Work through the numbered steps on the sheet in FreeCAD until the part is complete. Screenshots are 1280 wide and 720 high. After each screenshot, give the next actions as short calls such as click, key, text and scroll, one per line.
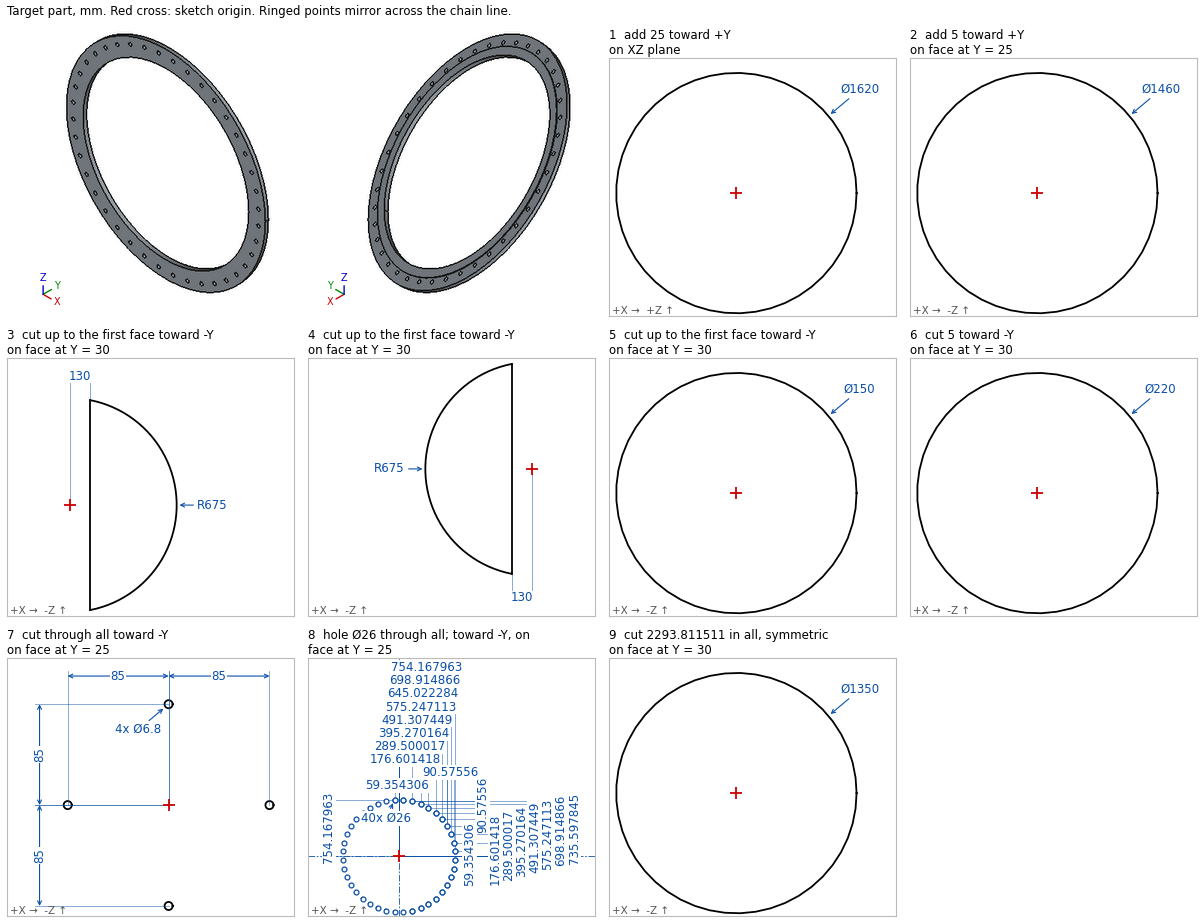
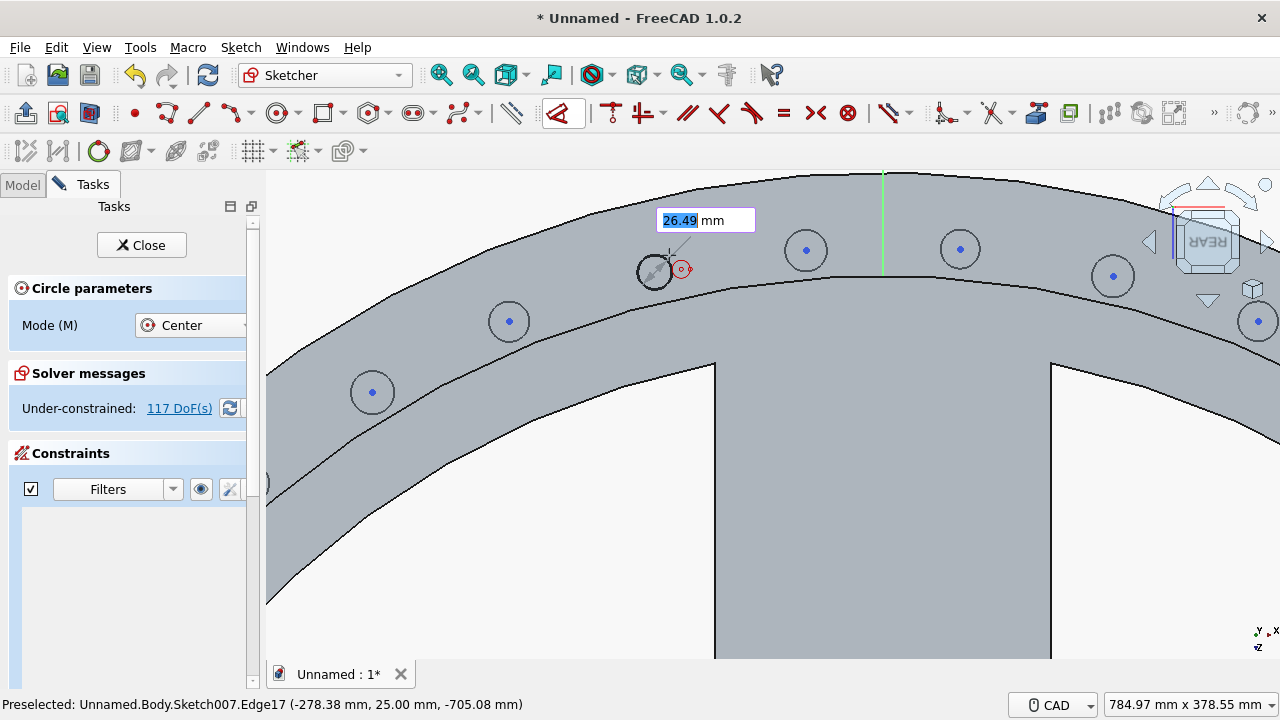
click(667, 257)
key(Escape)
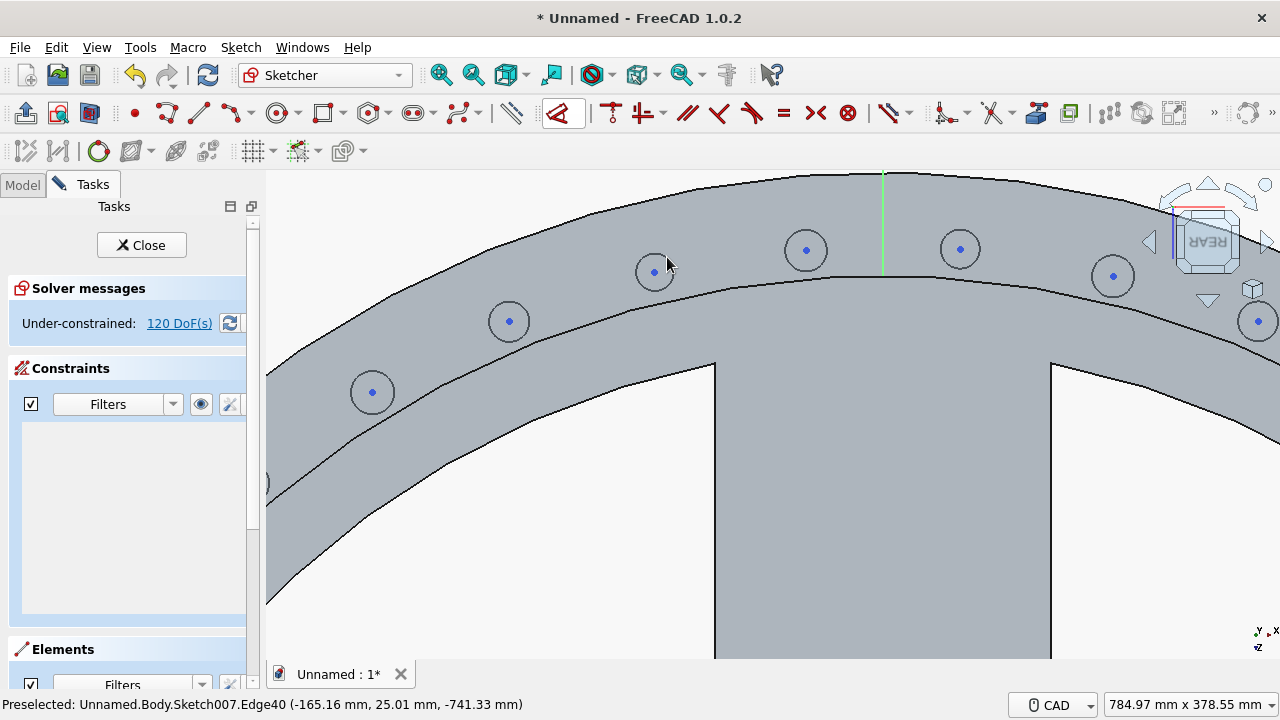
click(821, 236)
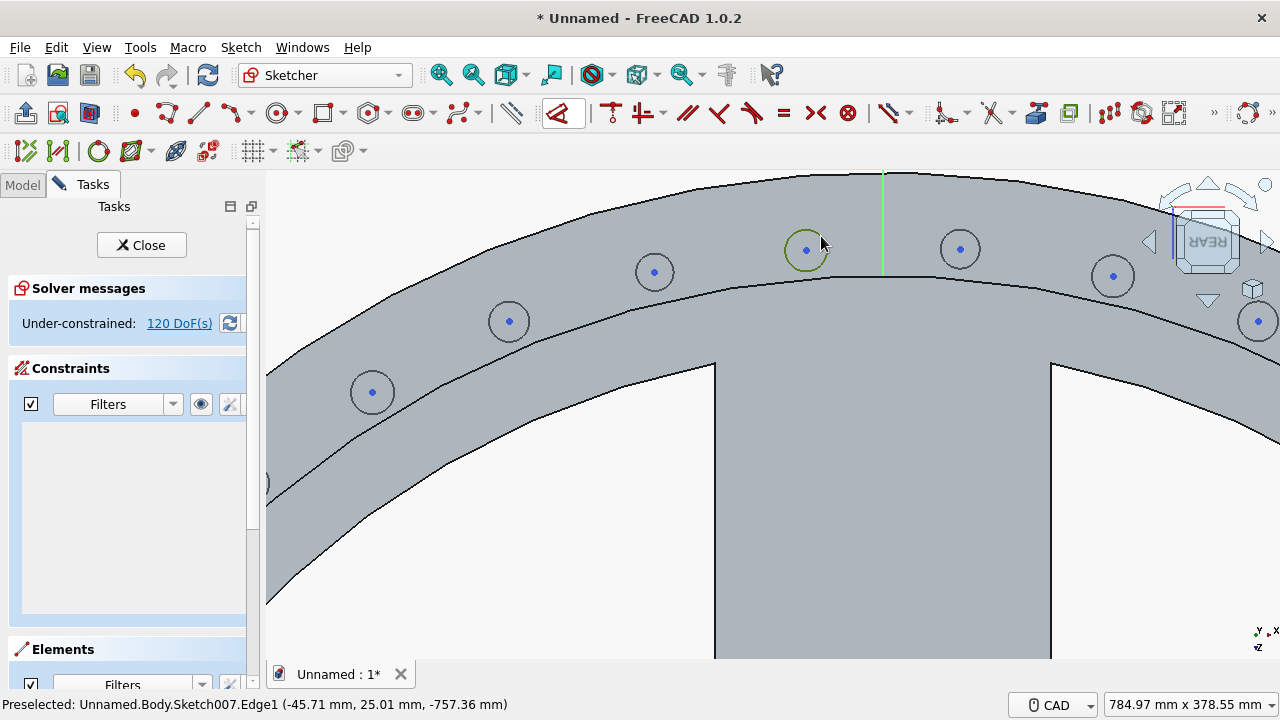
click(974, 235)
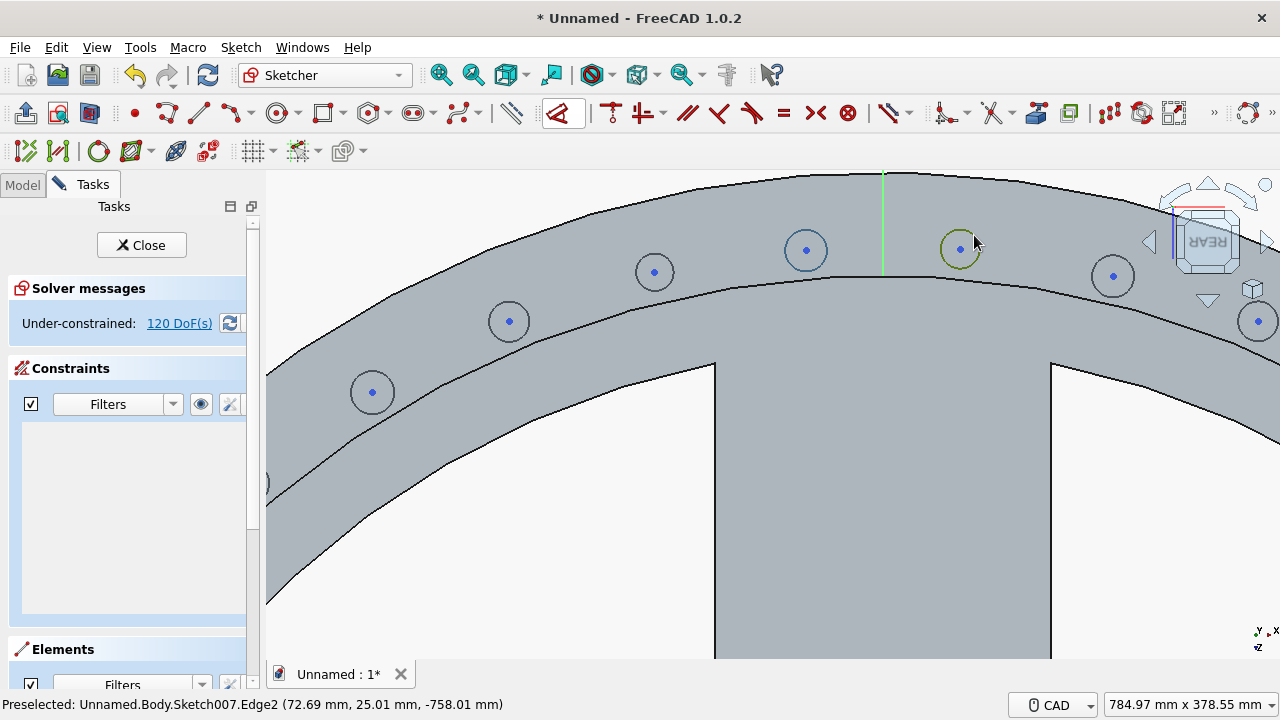
click(1098, 262)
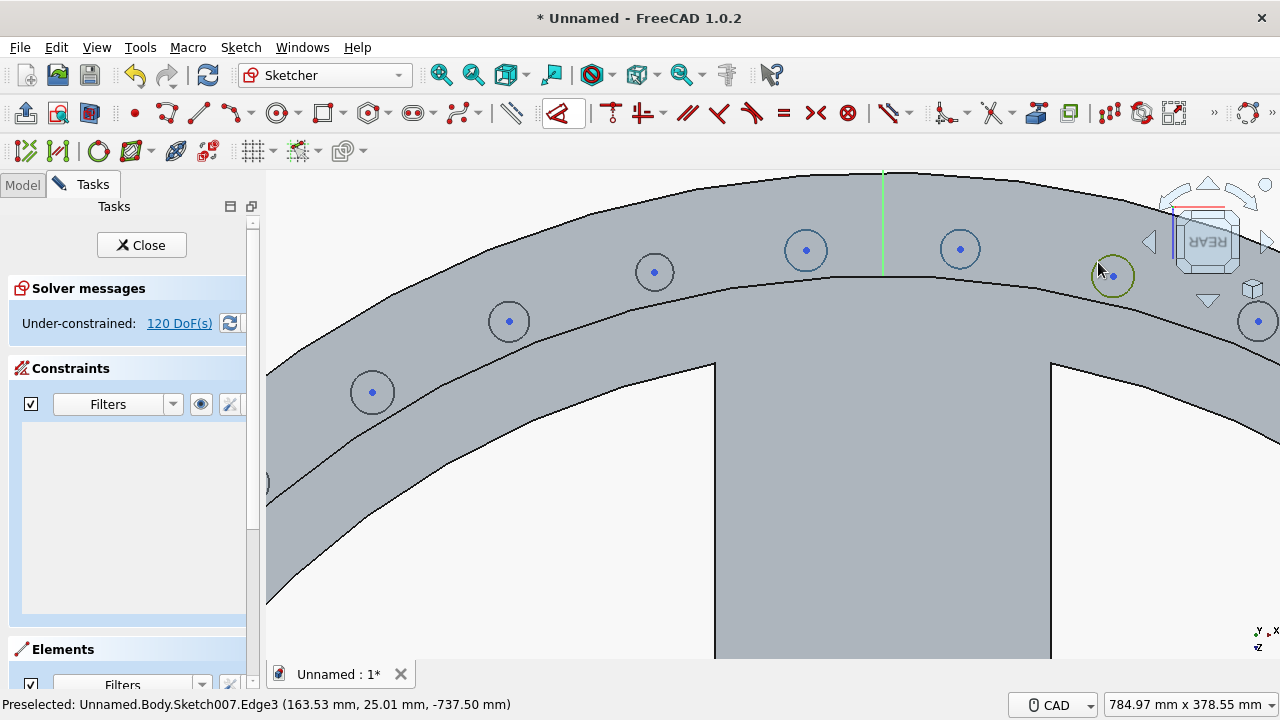
scroll(669, 255, down, 9)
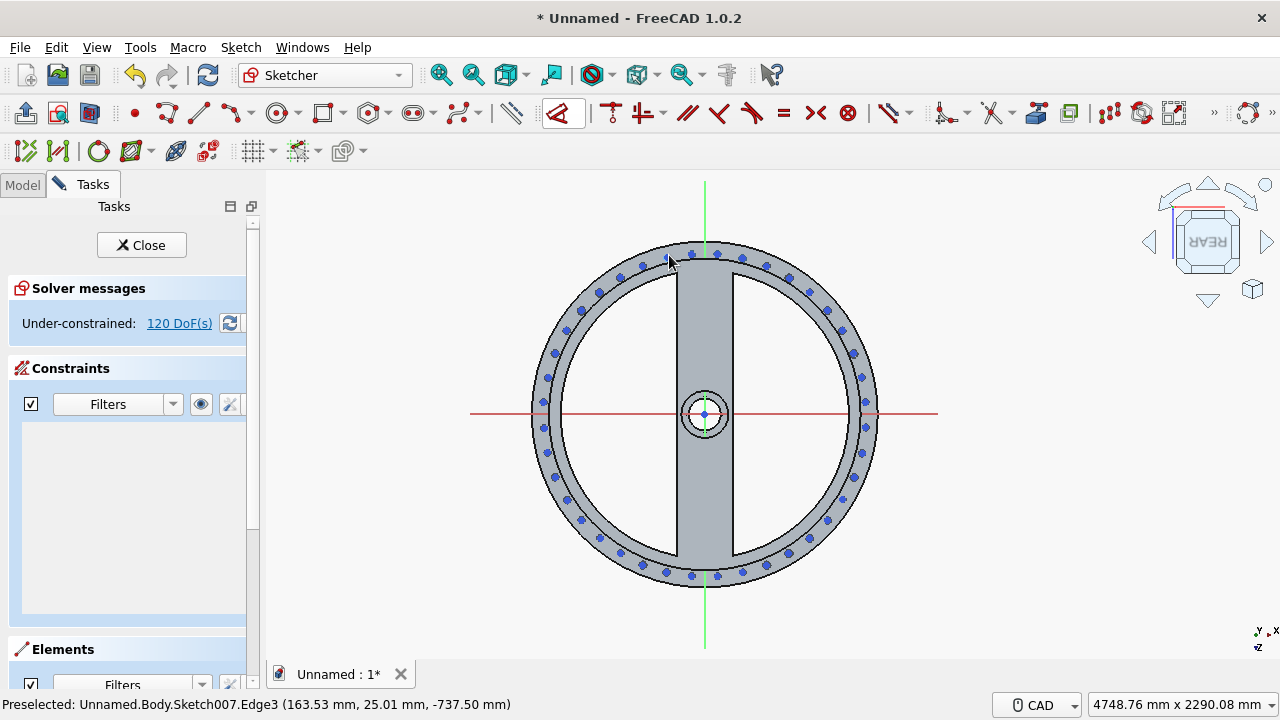
scroll(769, 264, up, 8)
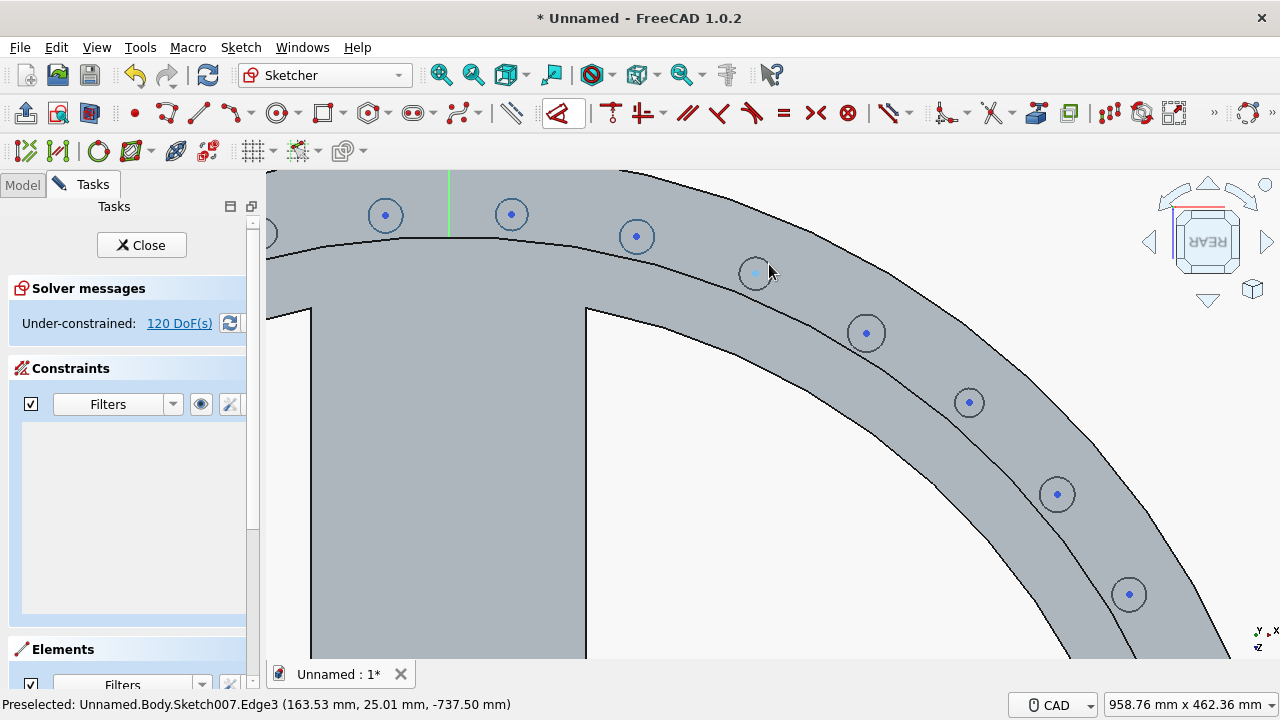
click(767, 262)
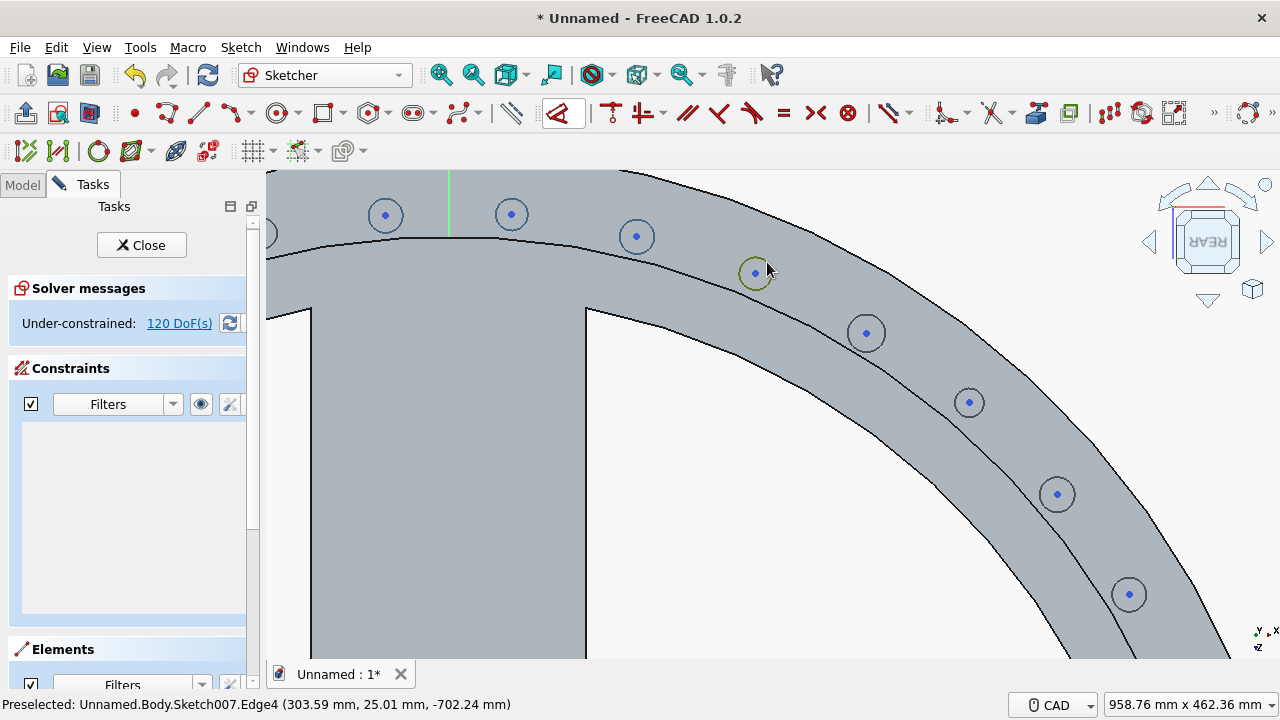
click(880, 320)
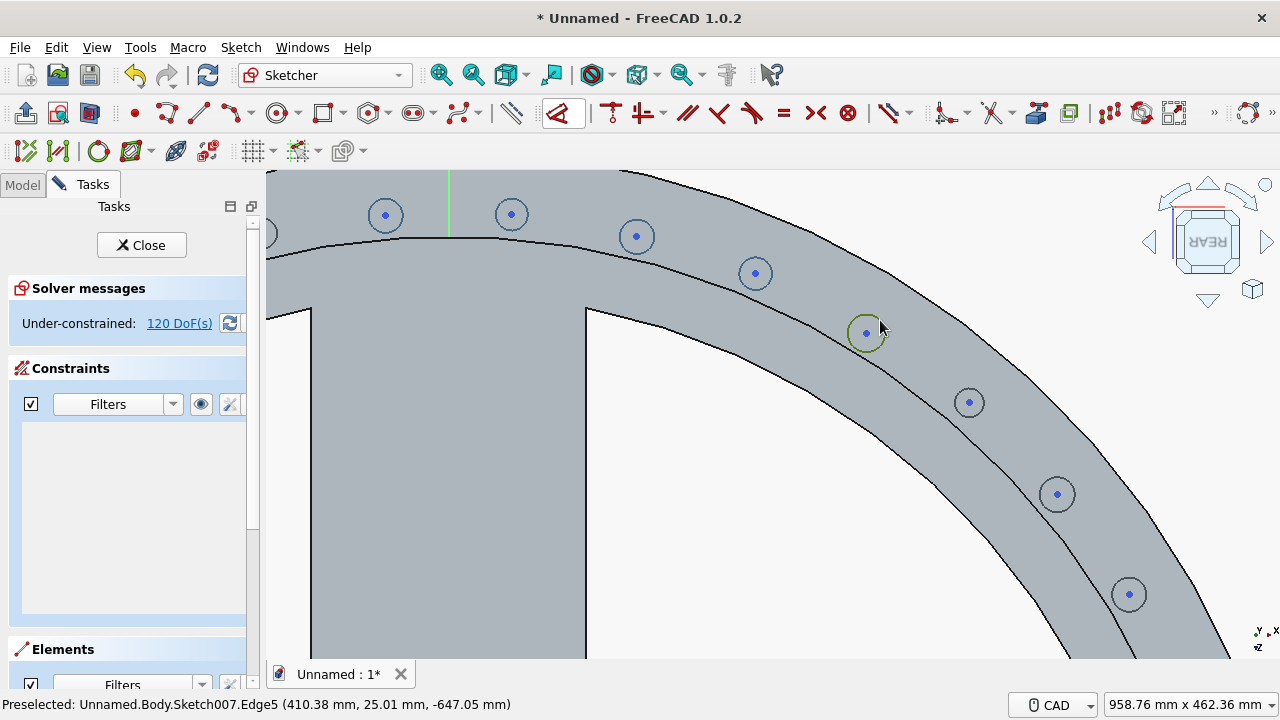
click(980, 393)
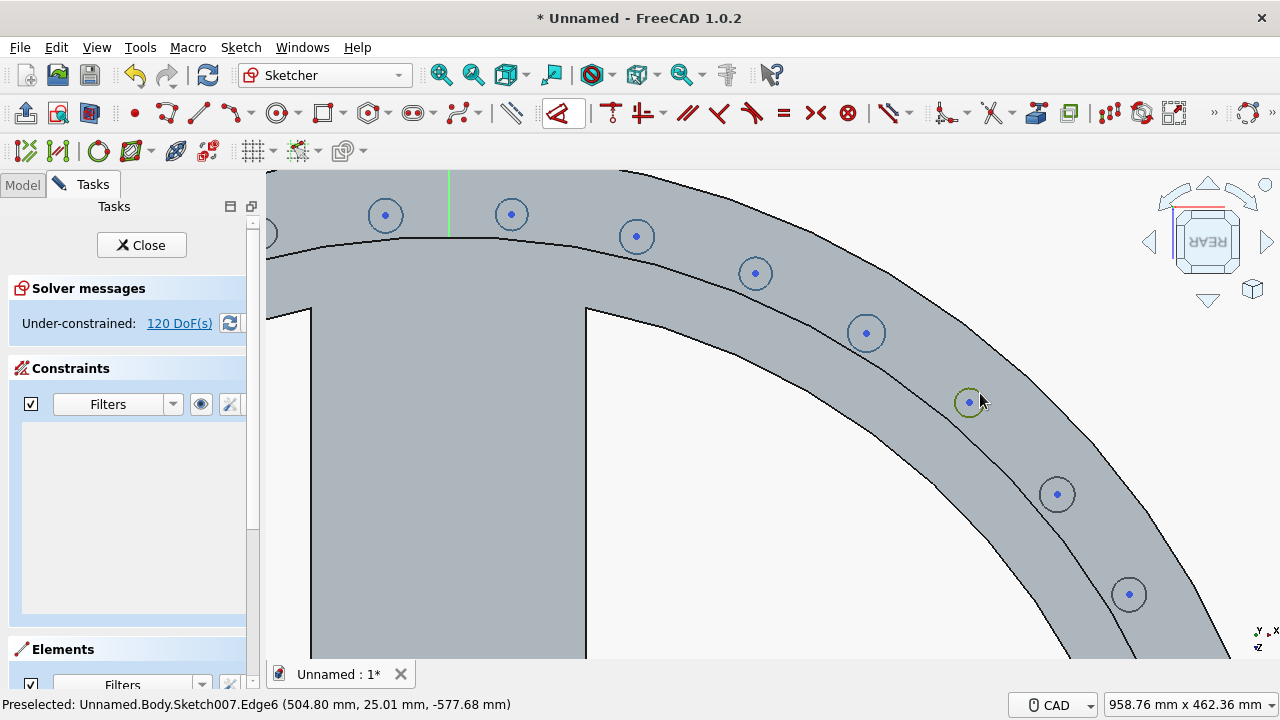
click(1070, 482)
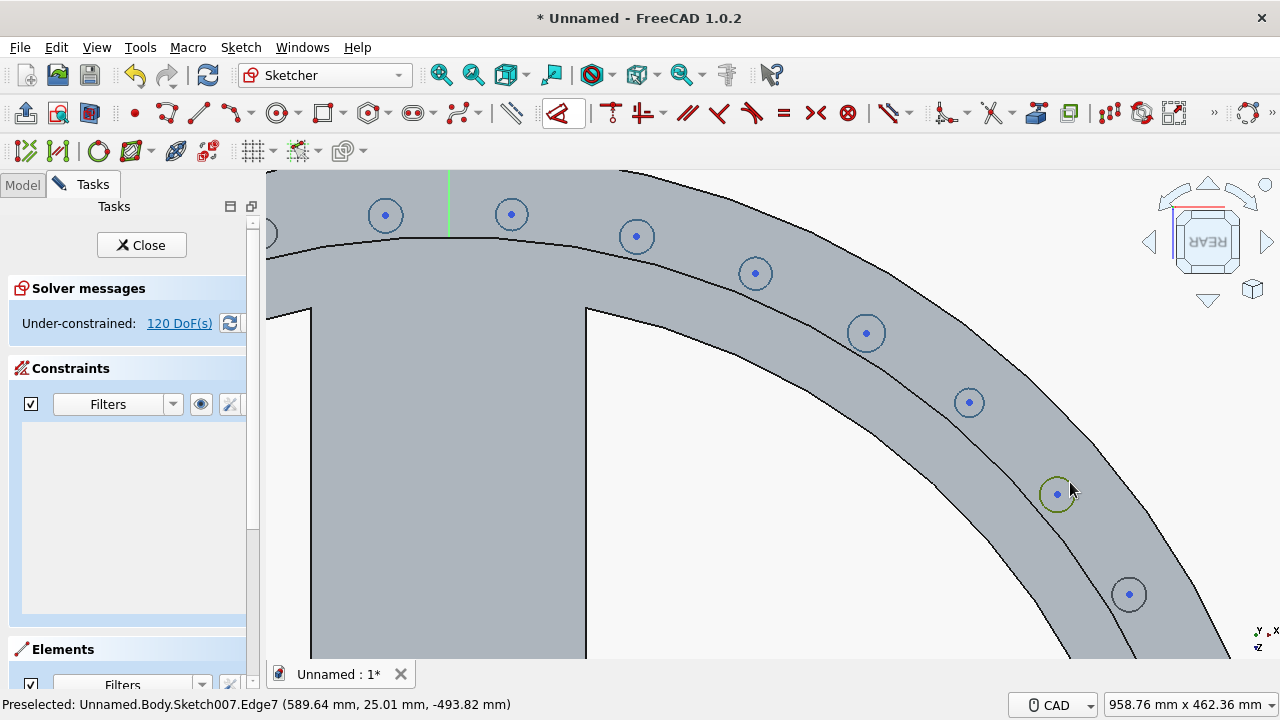
click(1112, 594)